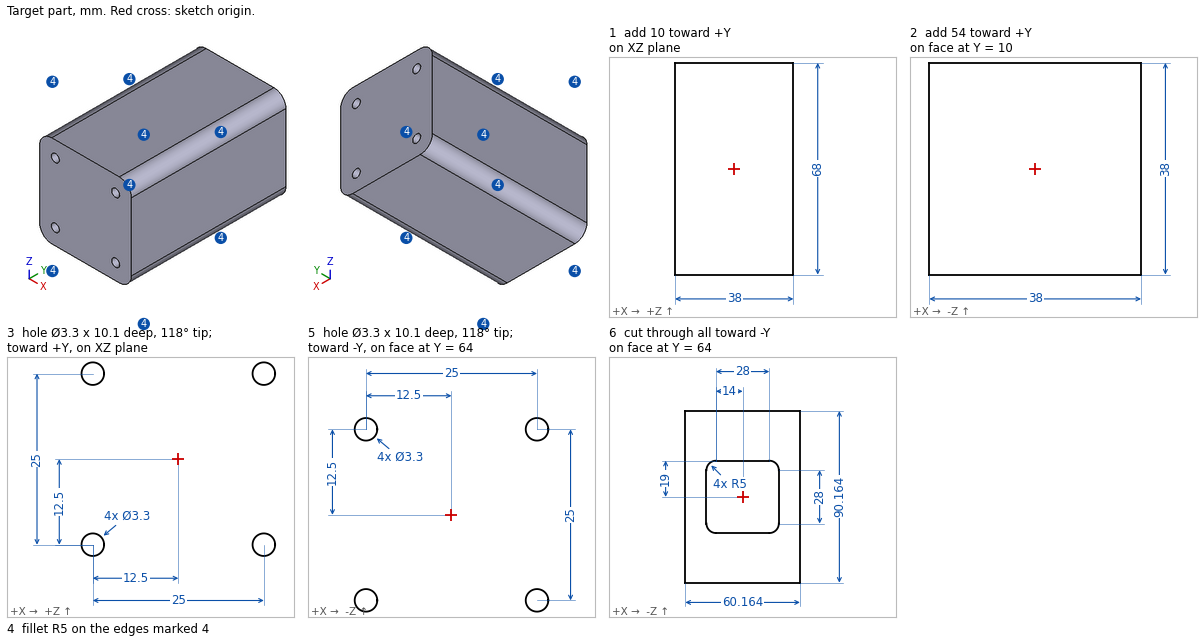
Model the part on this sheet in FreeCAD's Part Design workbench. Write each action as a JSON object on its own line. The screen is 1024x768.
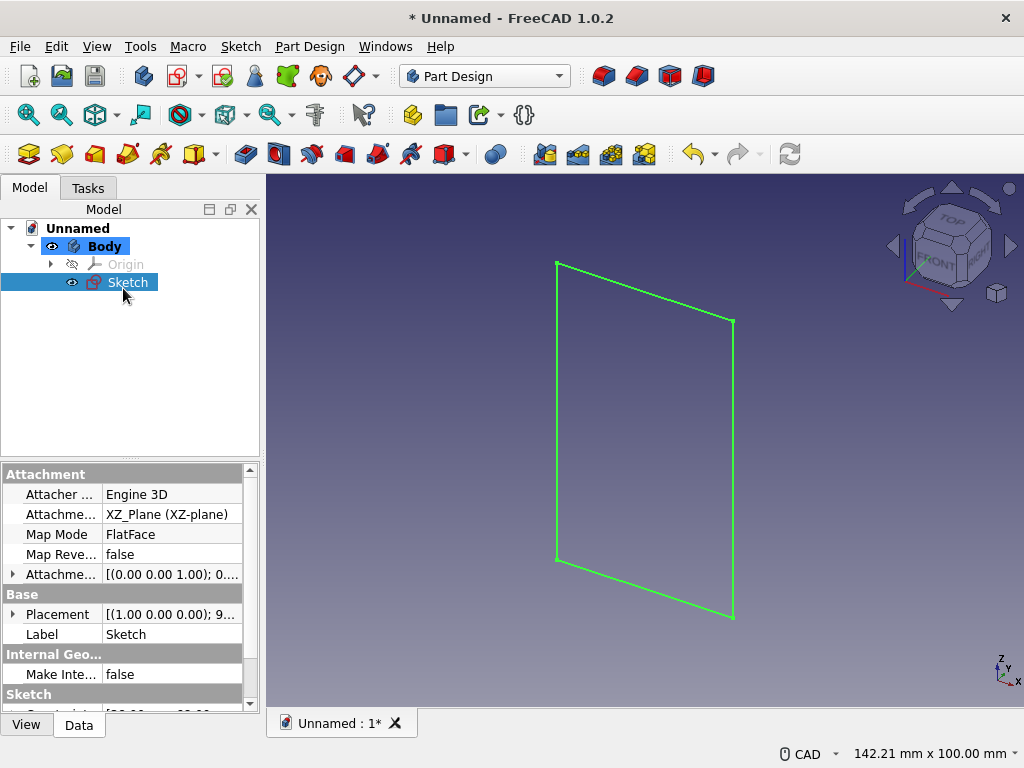
{"action": "left_click", "coordinate": [29, 154]}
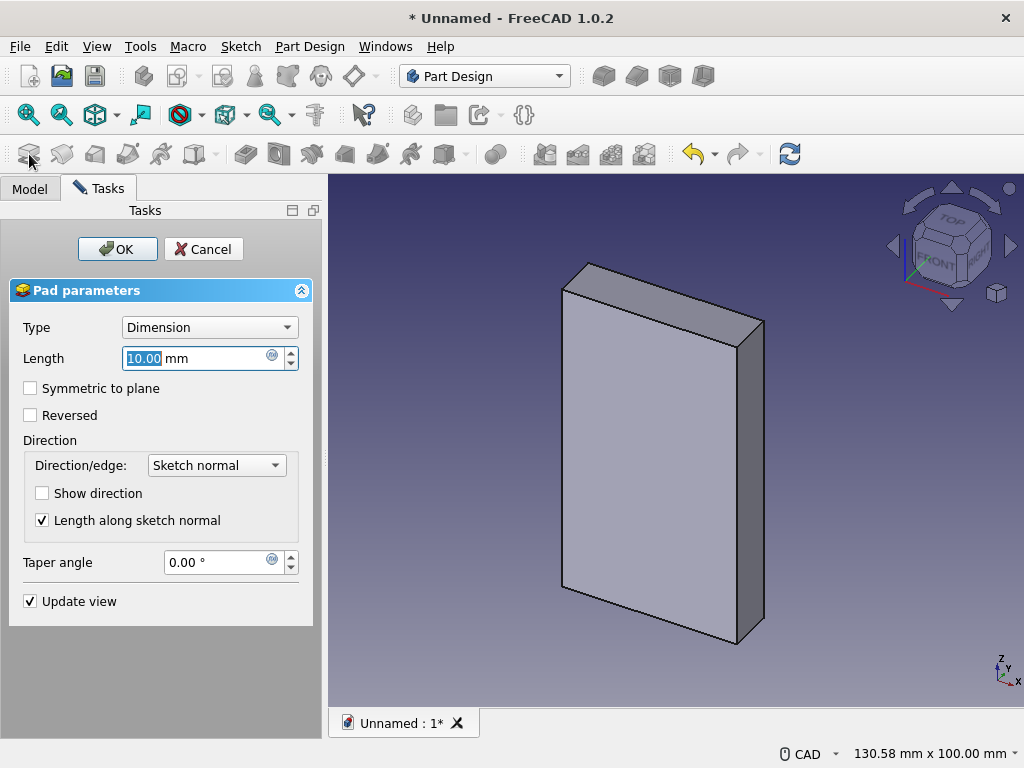
{"action": "type", "text": "10"}
{"action": "key", "text": "Tab"}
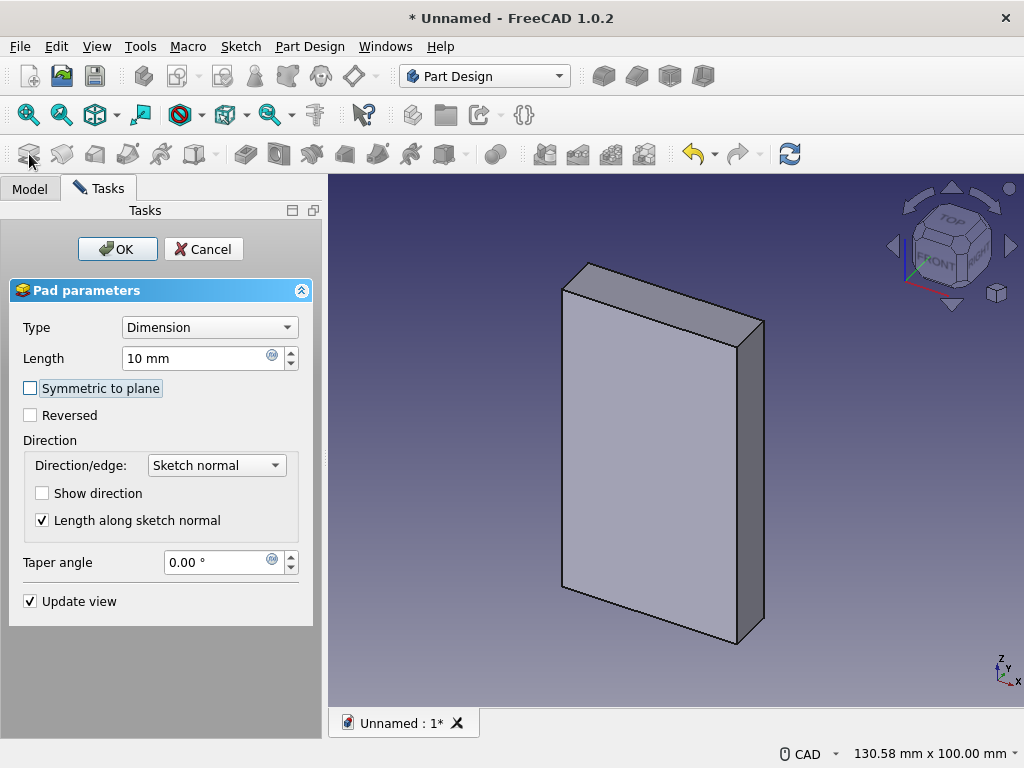
{"action": "left_click", "coordinate": [31, 415]}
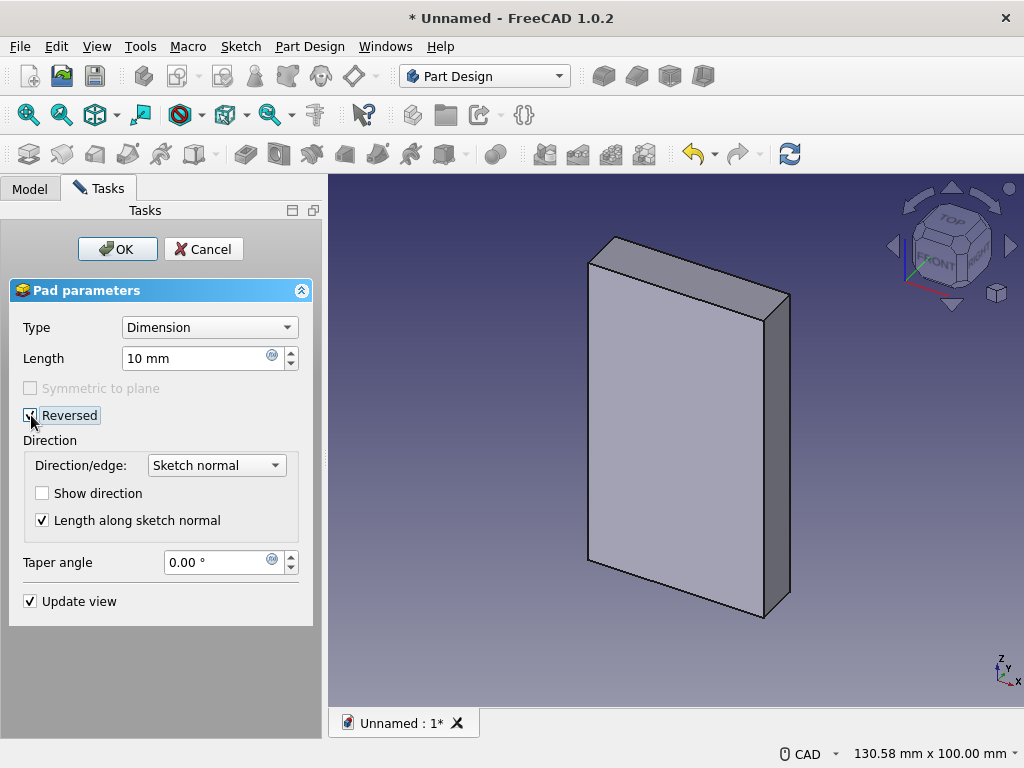
{"action": "left_click", "coordinate": [118, 249]}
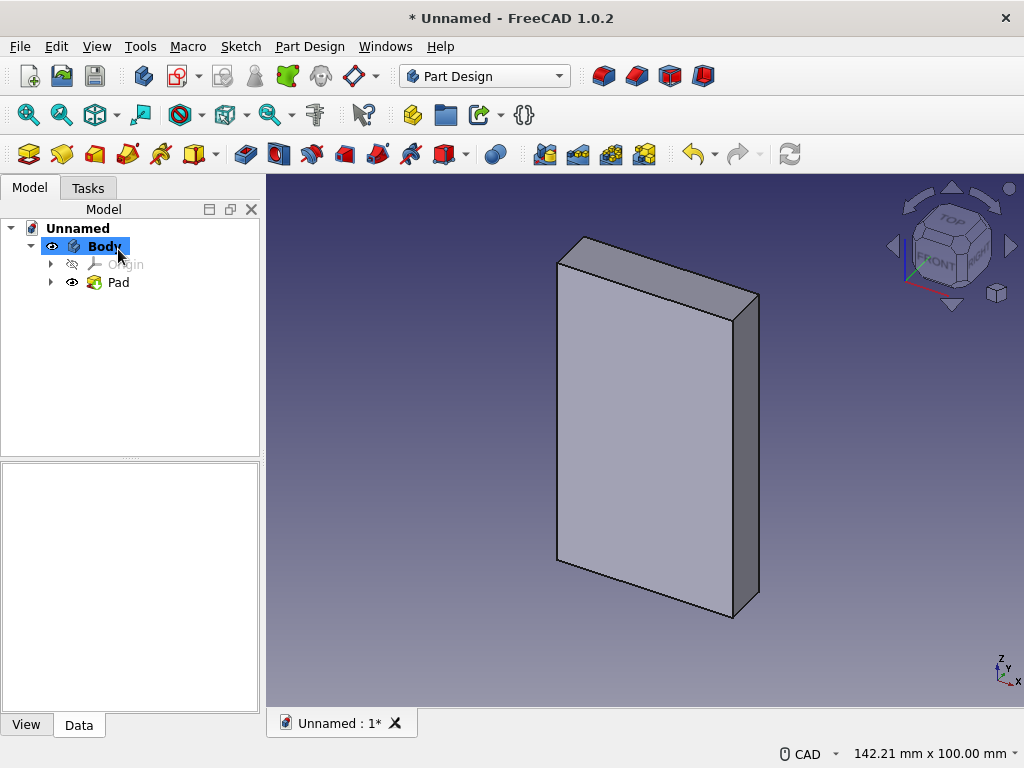
{"action": "key", "text": "4"}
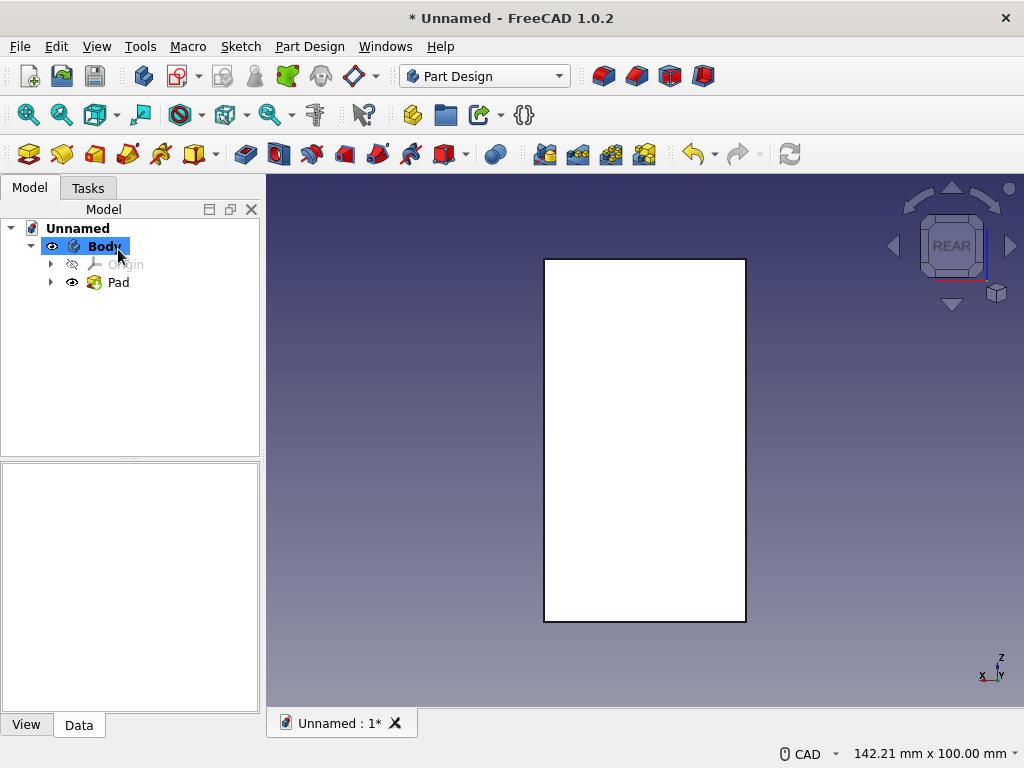
{"action": "left_click", "coordinate": [645, 388]}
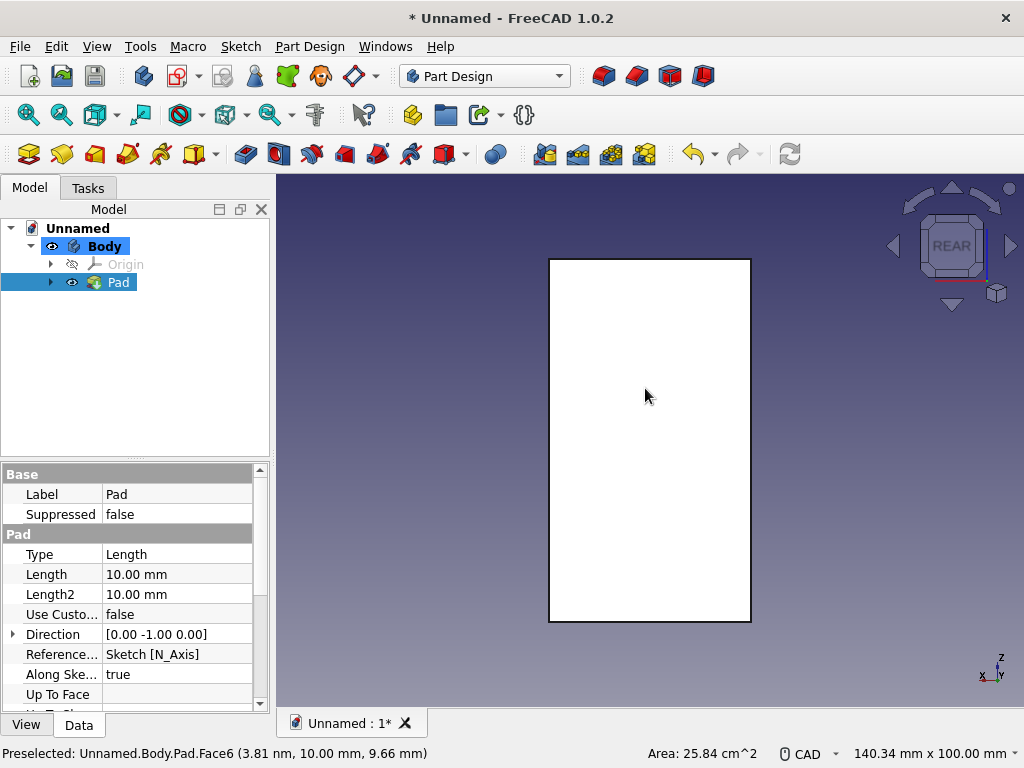
{"action": "left_click", "coordinate": [176, 76]}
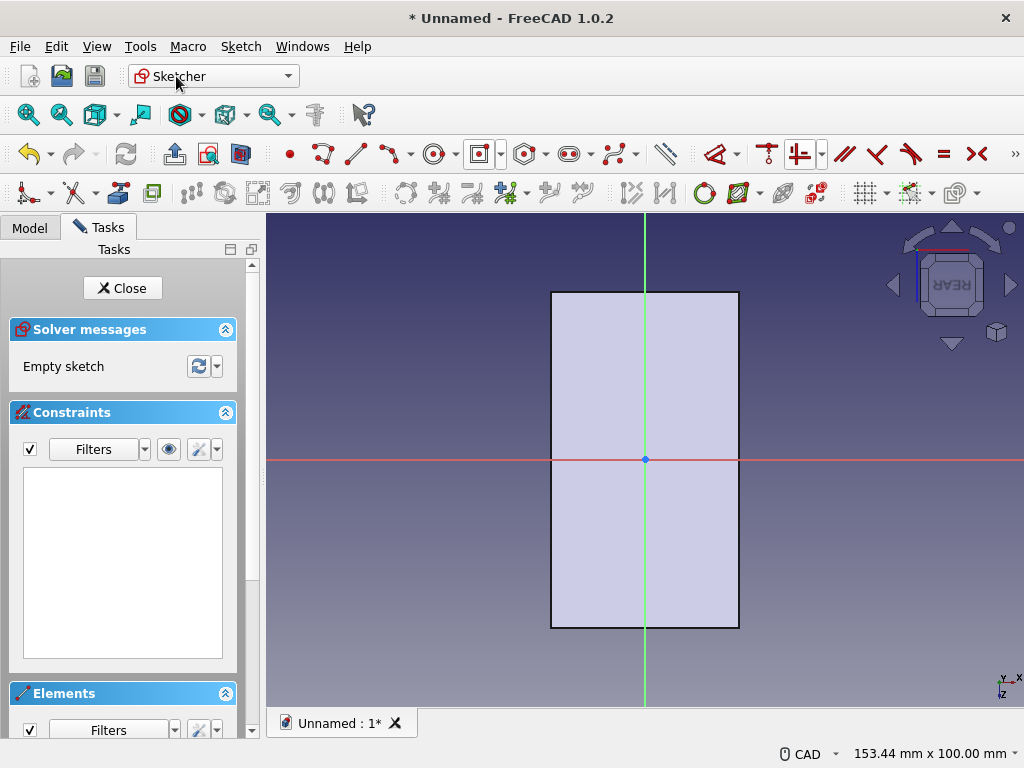
{"action": "scroll", "coordinate": [784, 460], "scroll_direction": "up", "scroll_amount": 2}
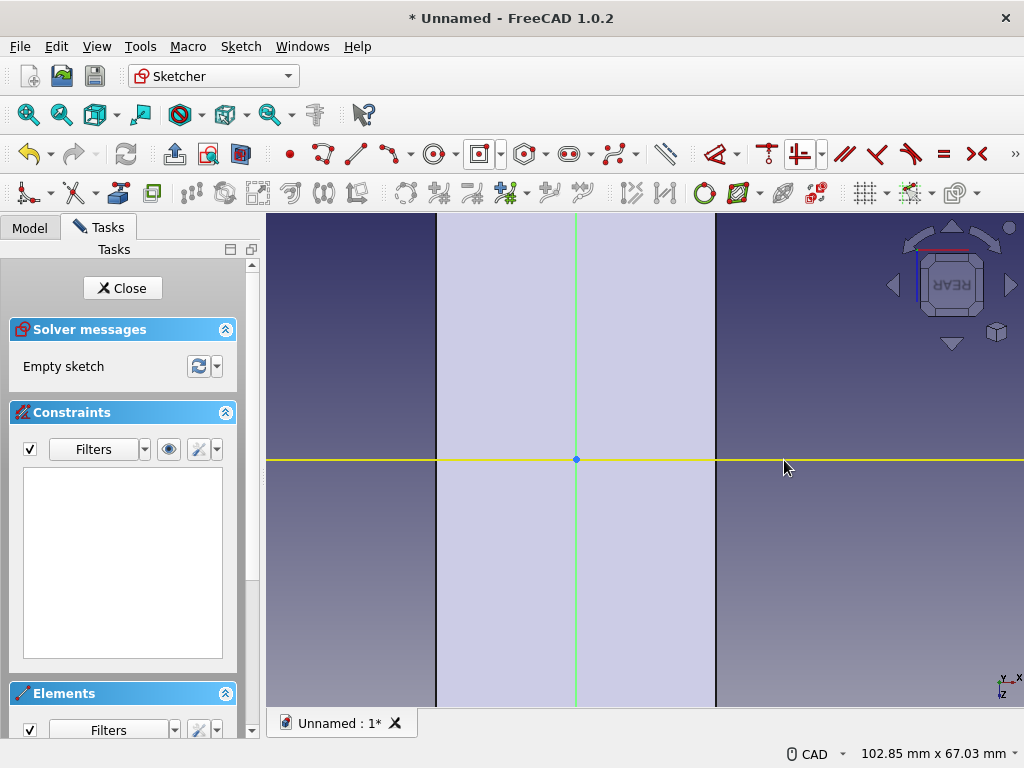
{"action": "left_click", "coordinate": [478, 154]}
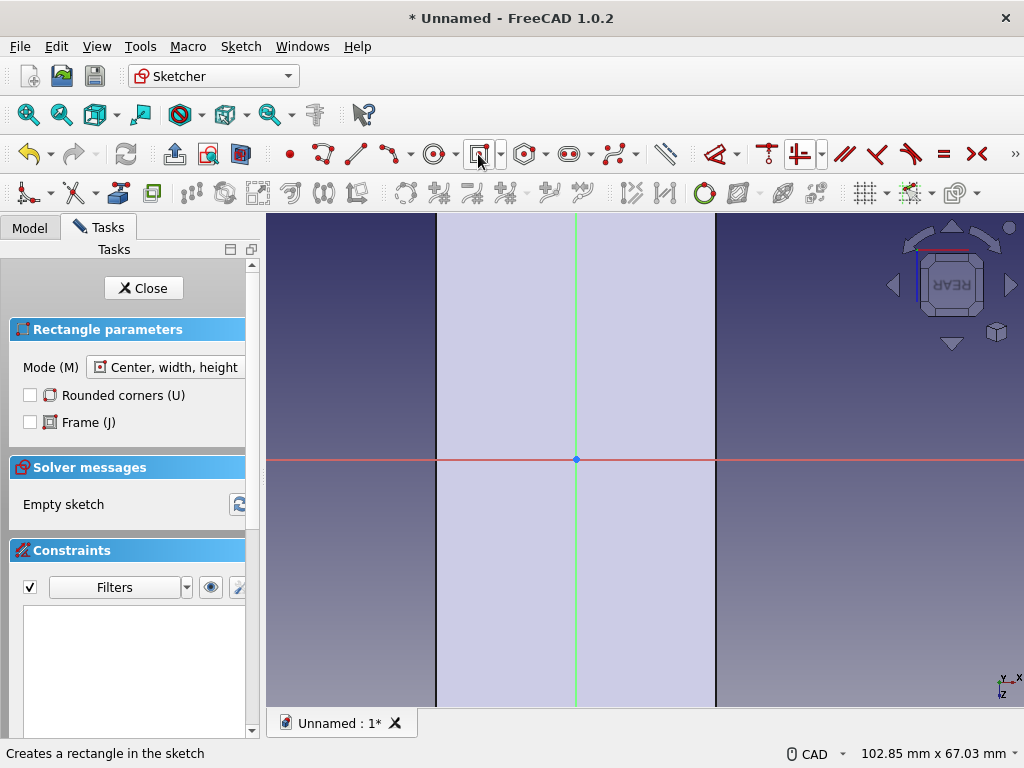
{"action": "left_click", "coordinate": [576, 460]}
{"action": "left_click", "coordinate": [716, 320]}
{"action": "key", "text": "Escape"}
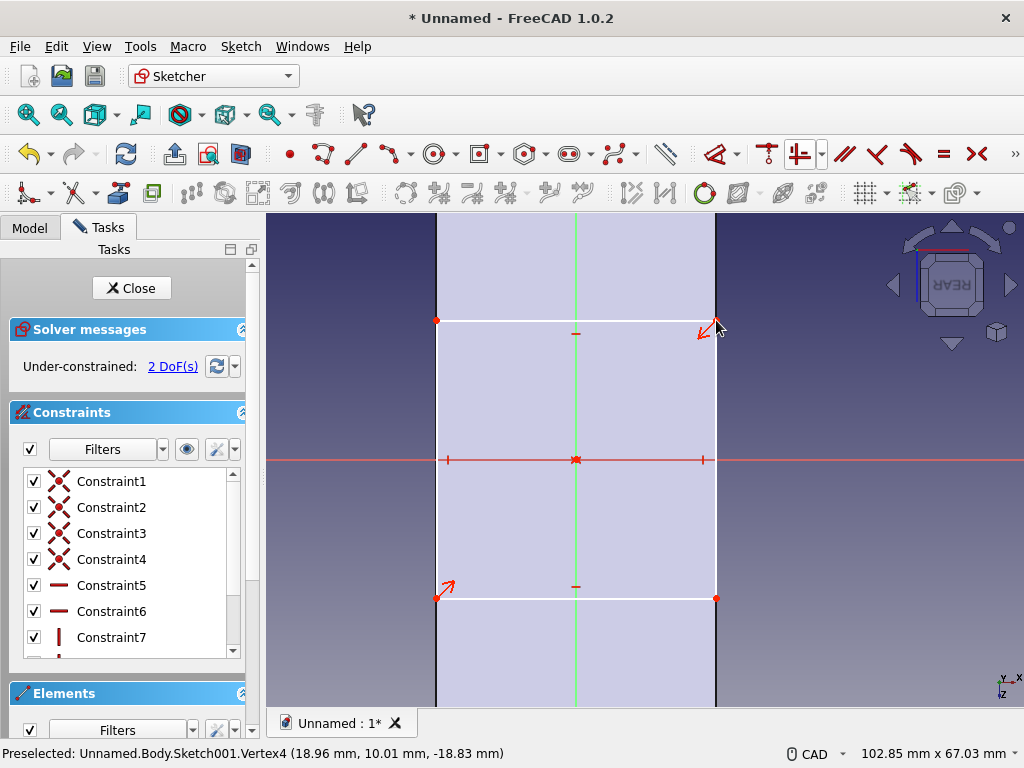
{"action": "left_click", "coordinate": [714, 154]}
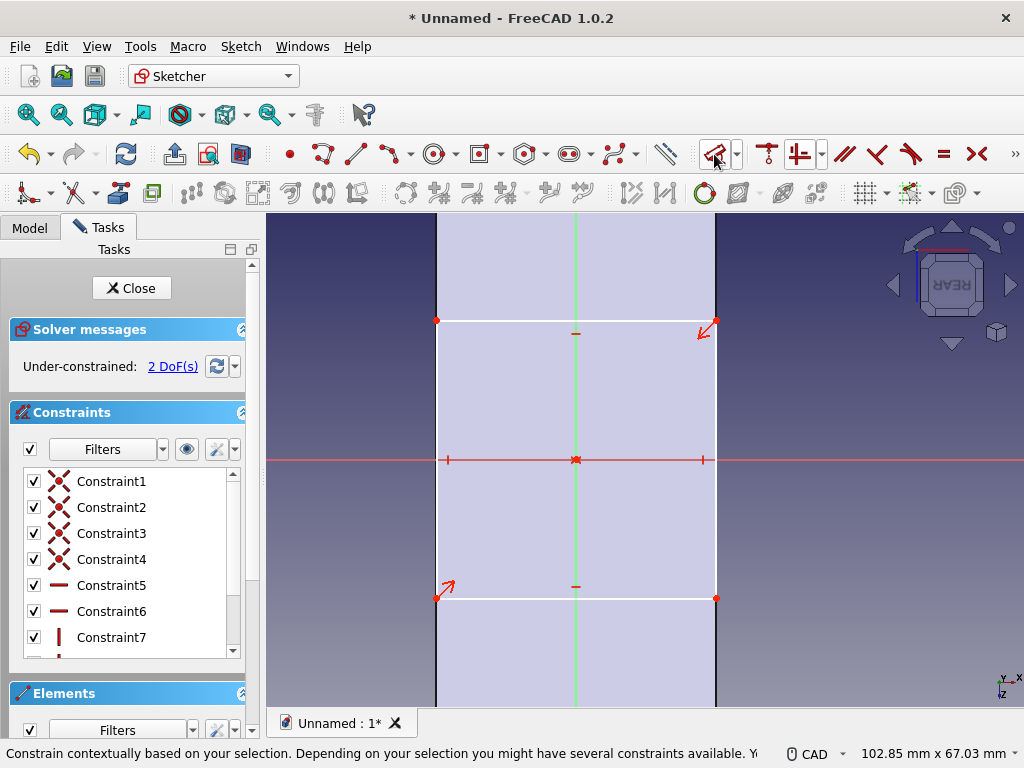
{"action": "left_click", "coordinate": [520, 599]}
{"action": "left_click", "coordinate": [512, 633]}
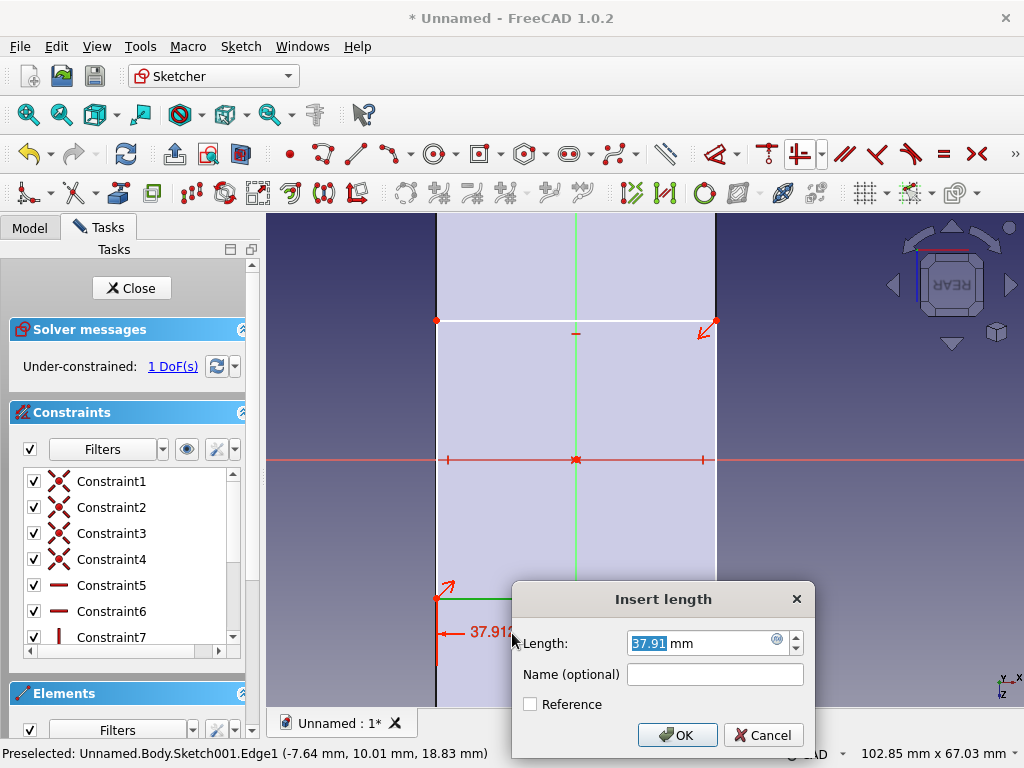
{"action": "type", "text": "38"}
{"action": "key", "text": "Return"}